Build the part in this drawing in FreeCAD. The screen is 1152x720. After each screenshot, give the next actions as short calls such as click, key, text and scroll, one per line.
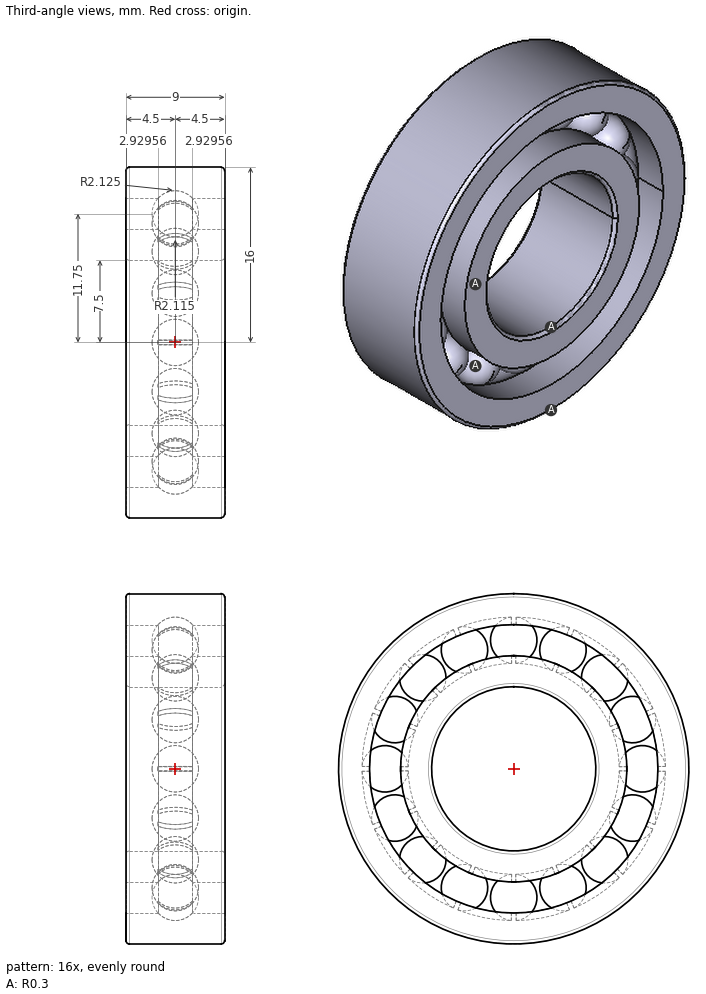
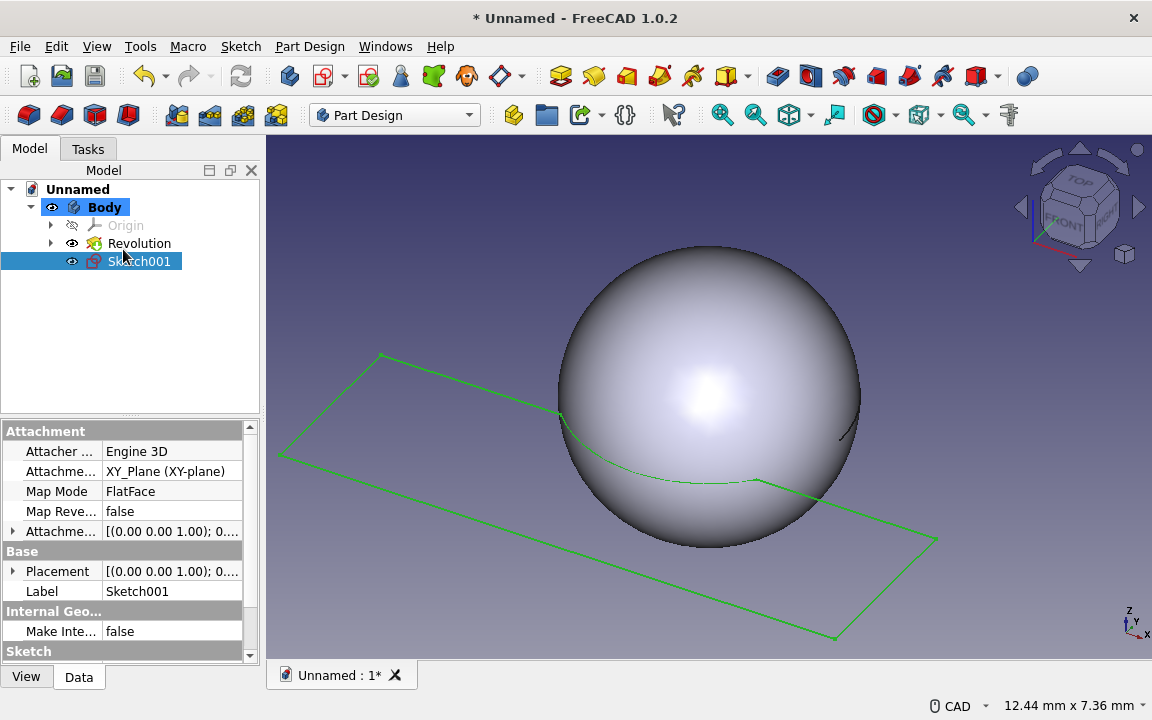
click(594, 76)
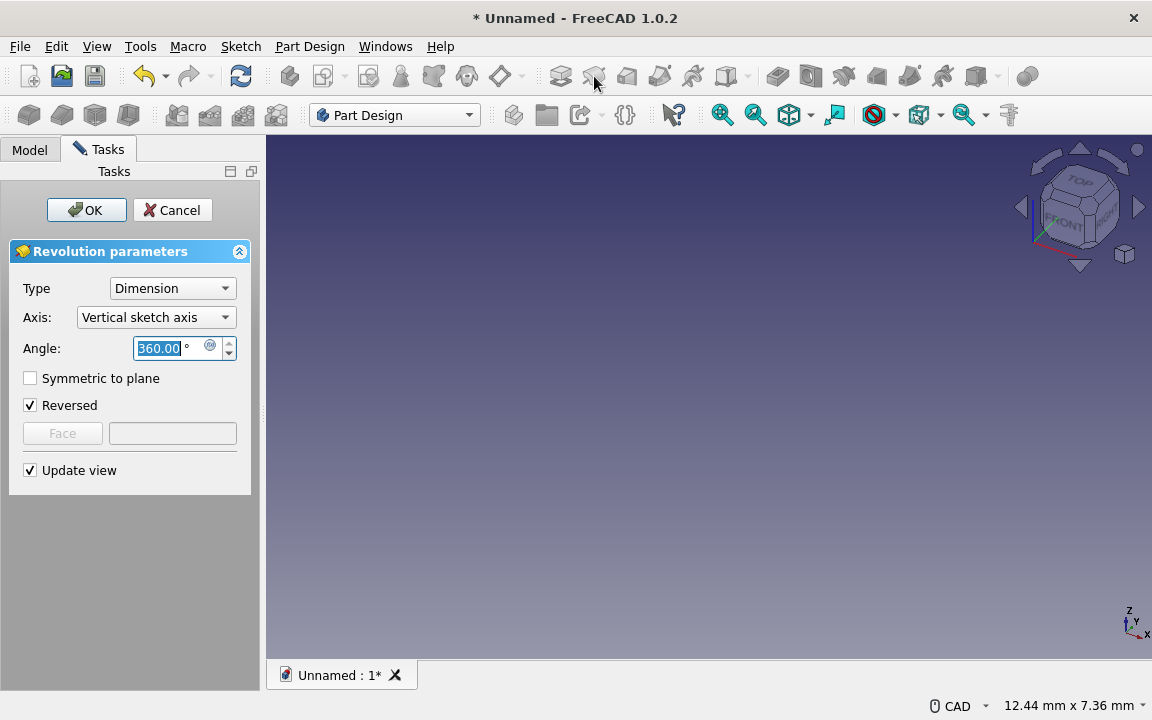
click(157, 318)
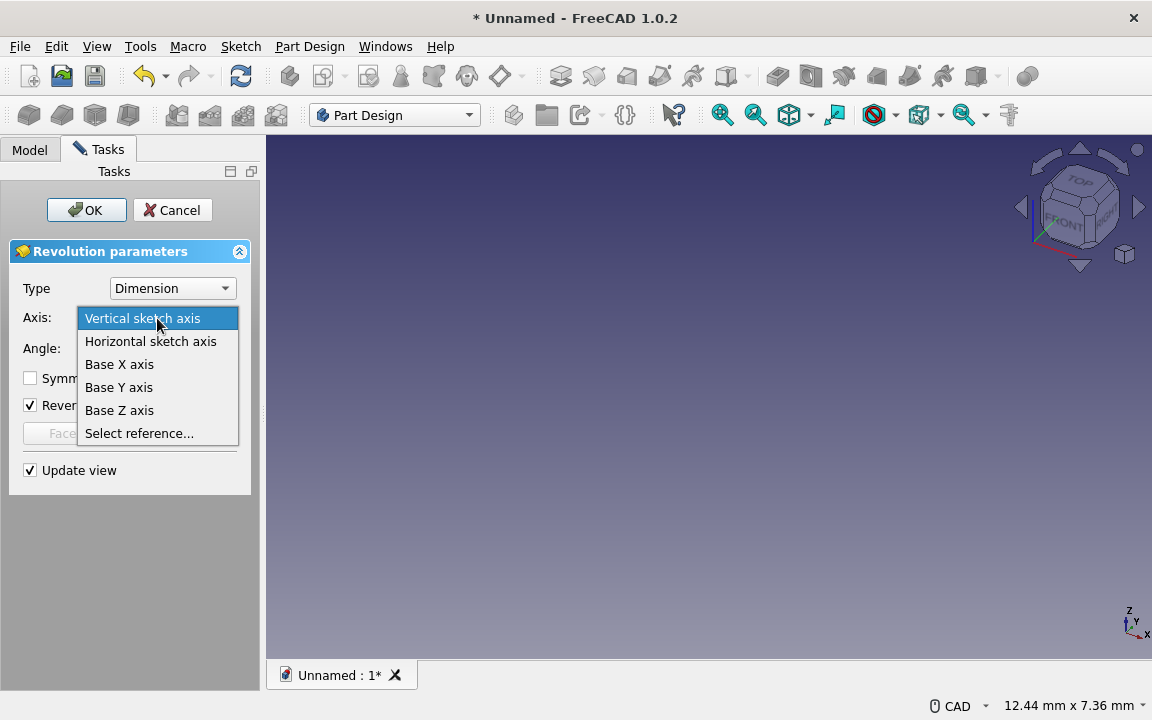
click(156, 342)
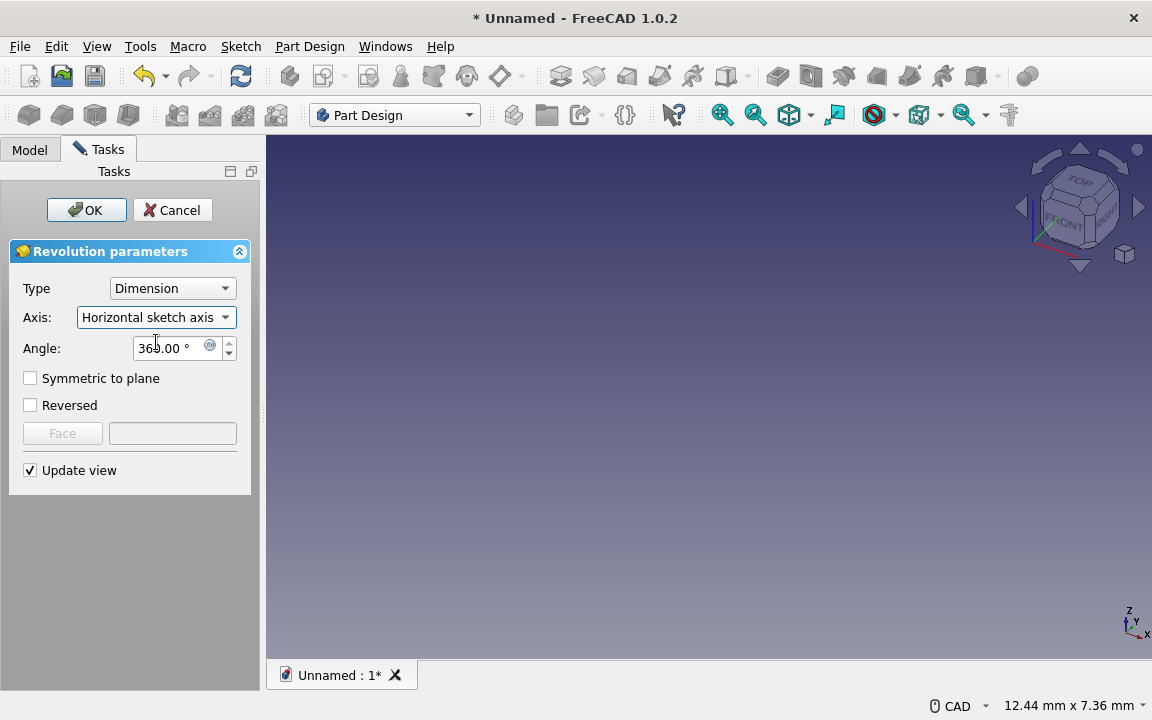
click(87, 210)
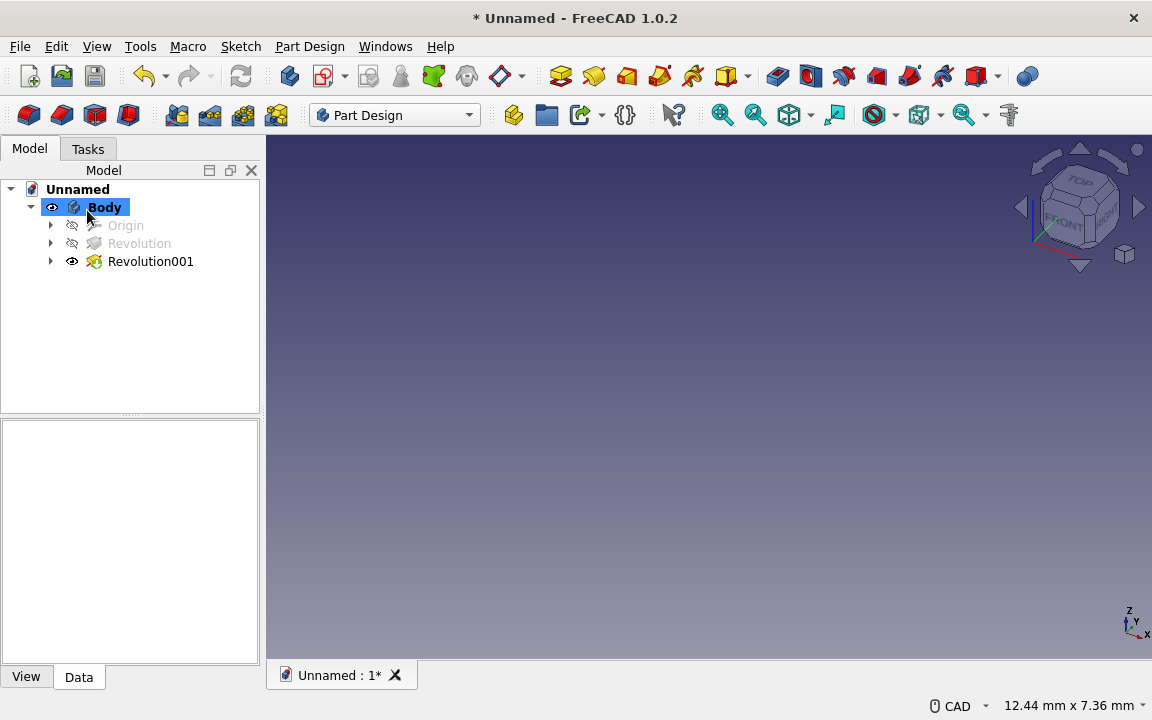
click(723, 116)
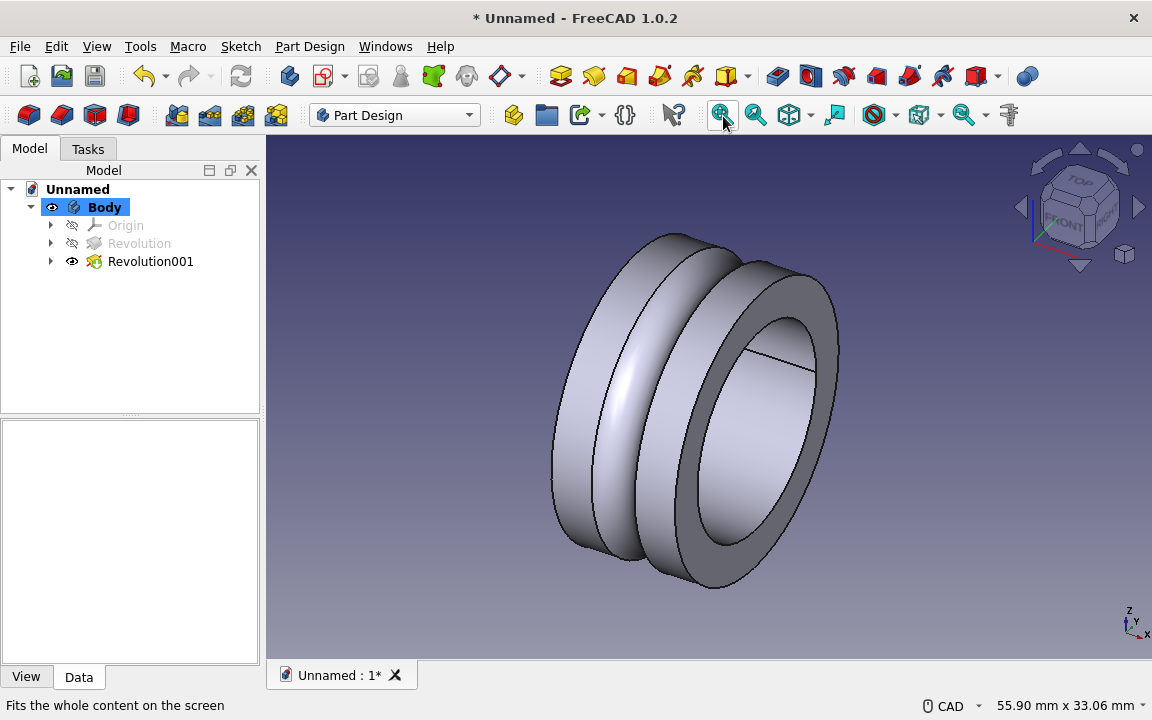
click(322, 76)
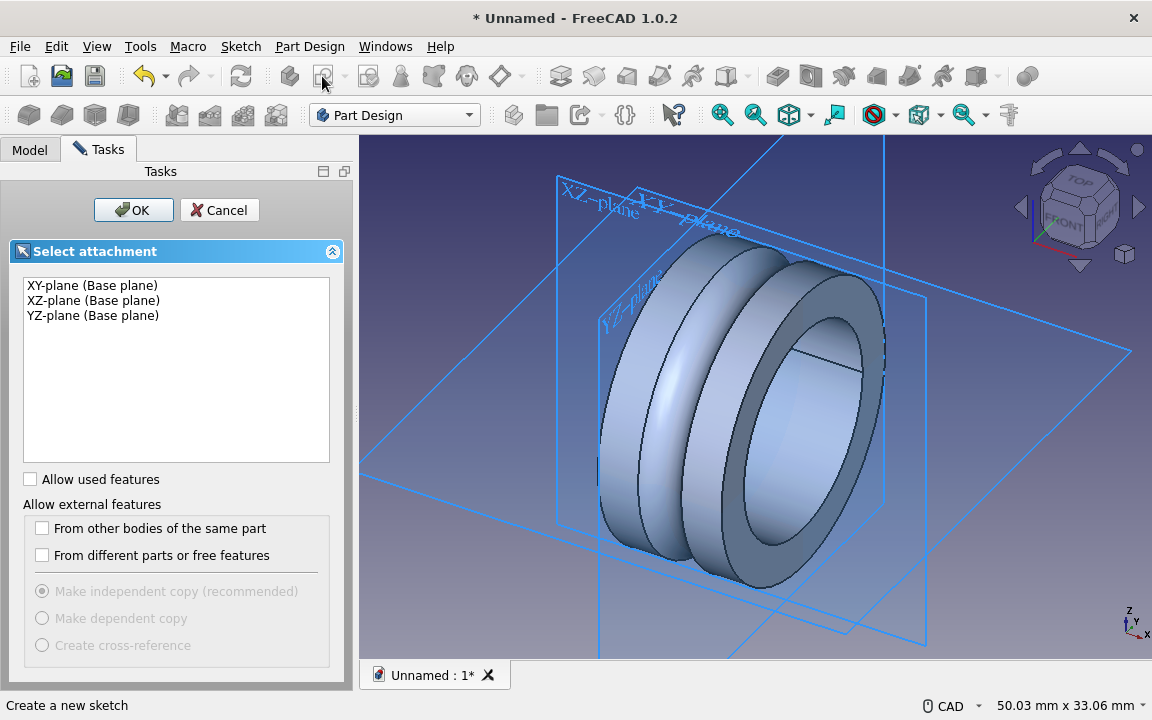
click(84, 286)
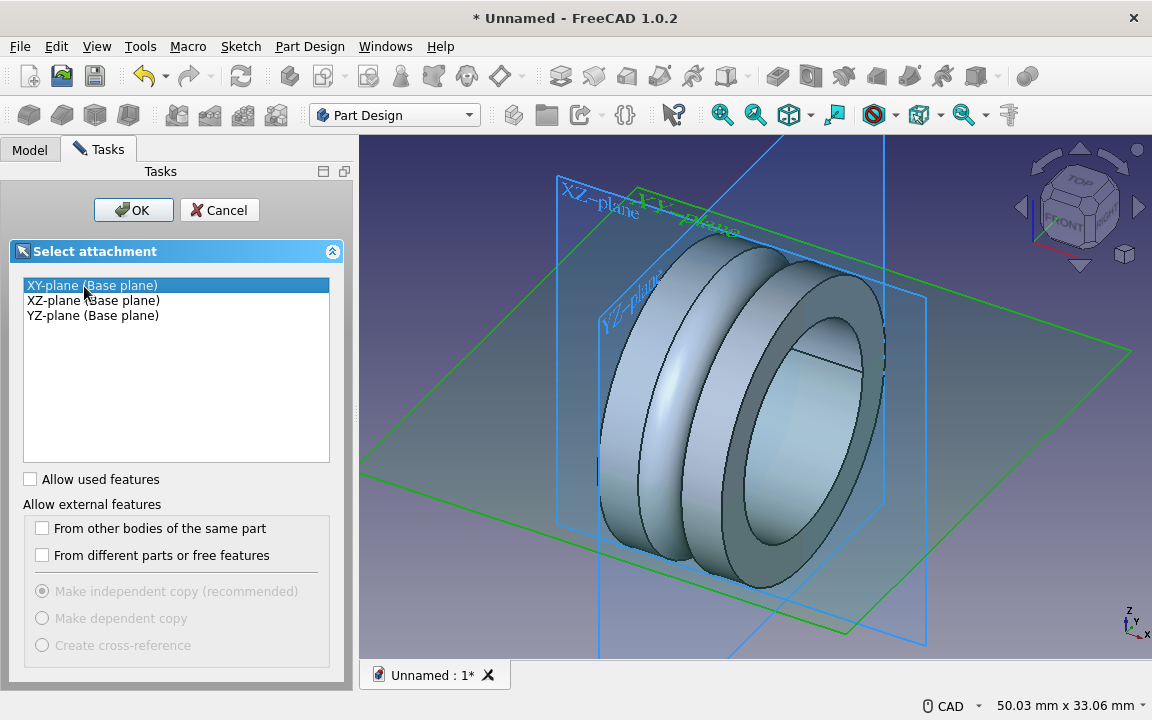
click(134, 210)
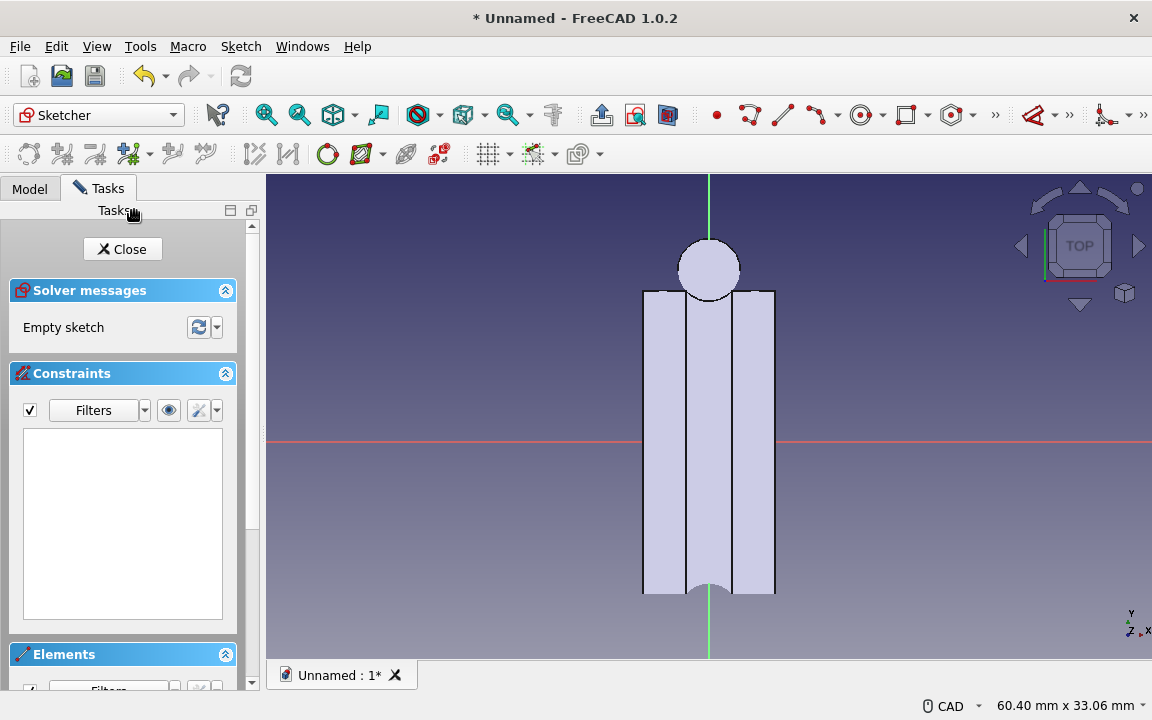
click(668, 116)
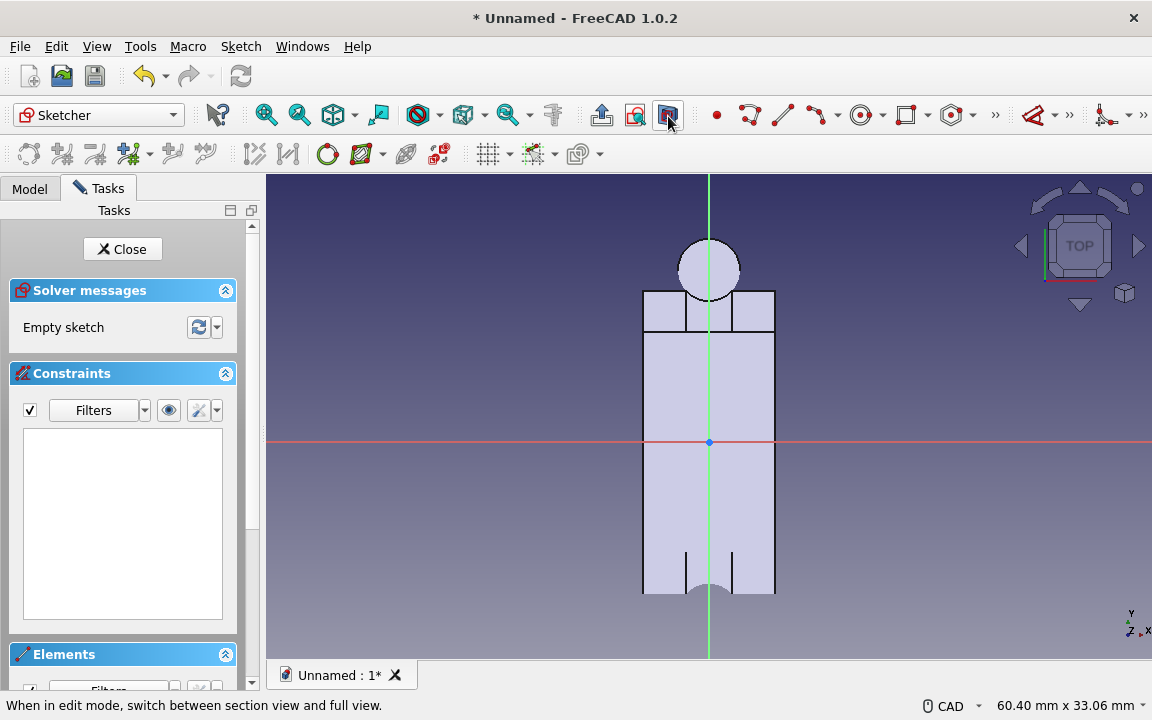
scroll(331, 631, down, 1)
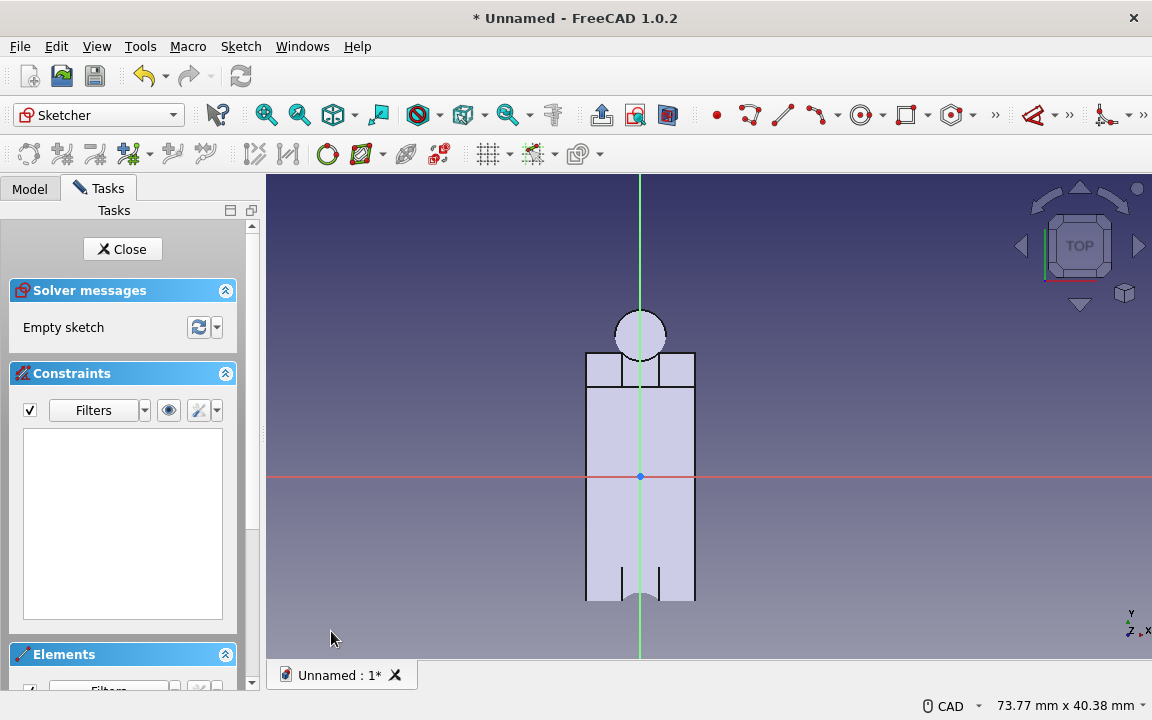
scroll(640, 308, up, 2)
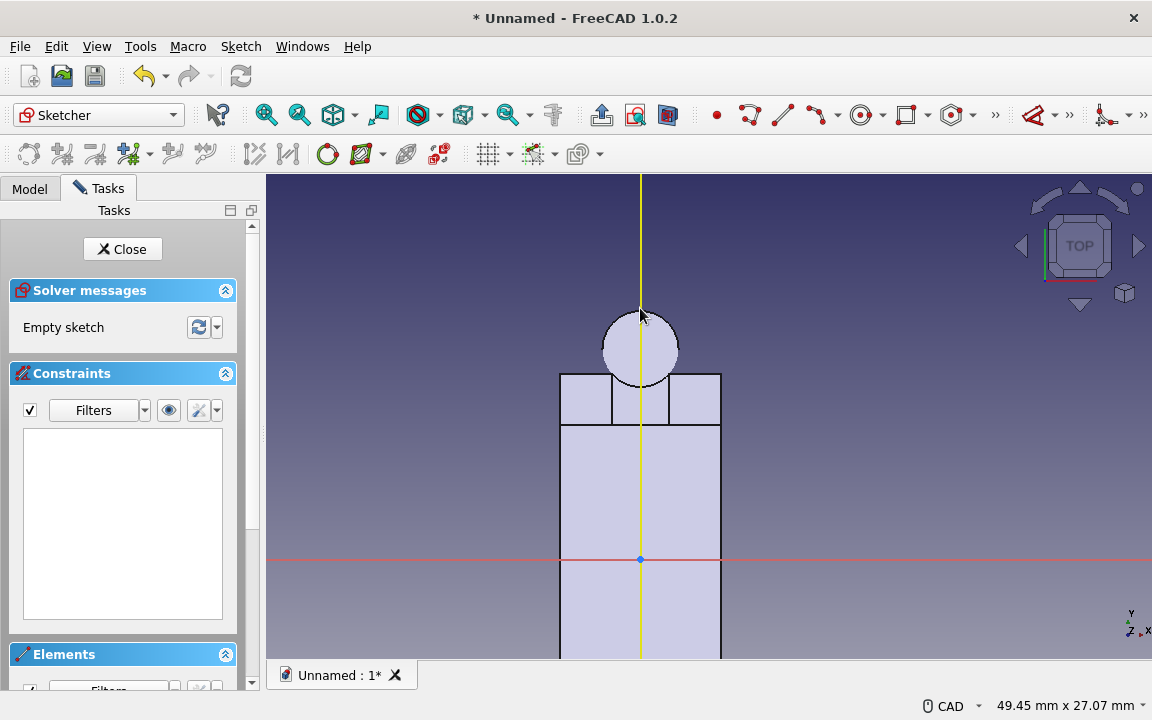
key(g)
key(m)